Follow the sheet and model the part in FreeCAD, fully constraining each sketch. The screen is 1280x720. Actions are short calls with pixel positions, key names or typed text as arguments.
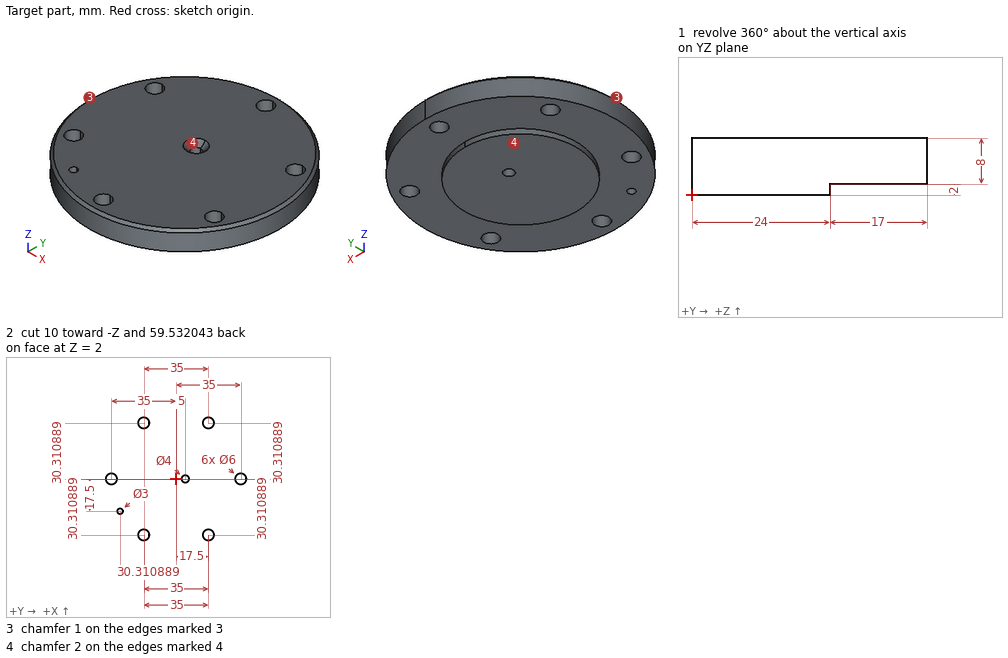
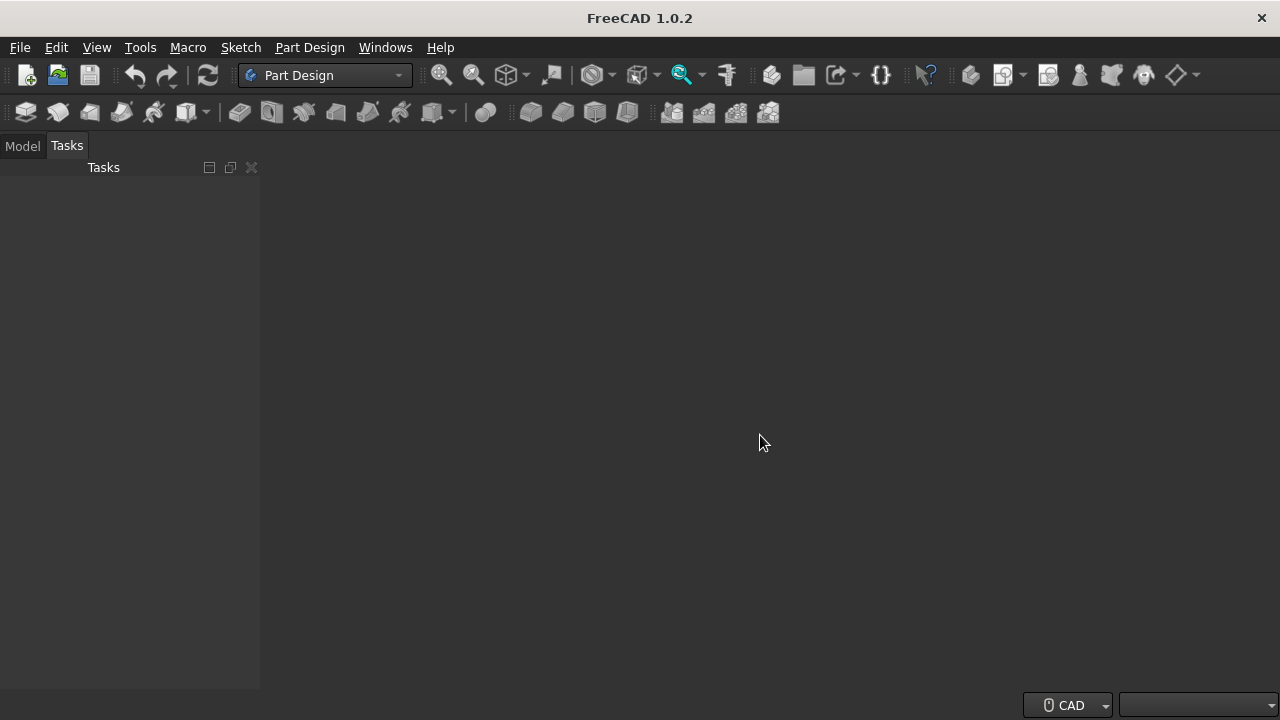
click(26, 76)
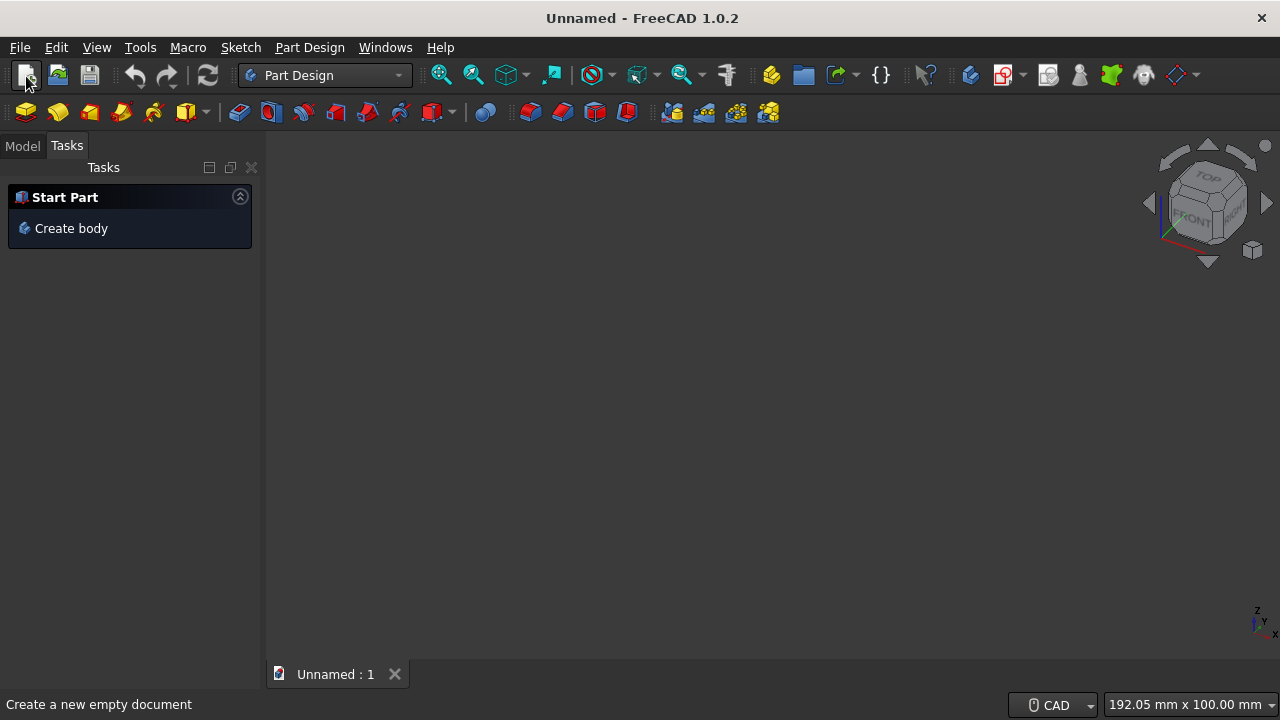
click(1004, 76)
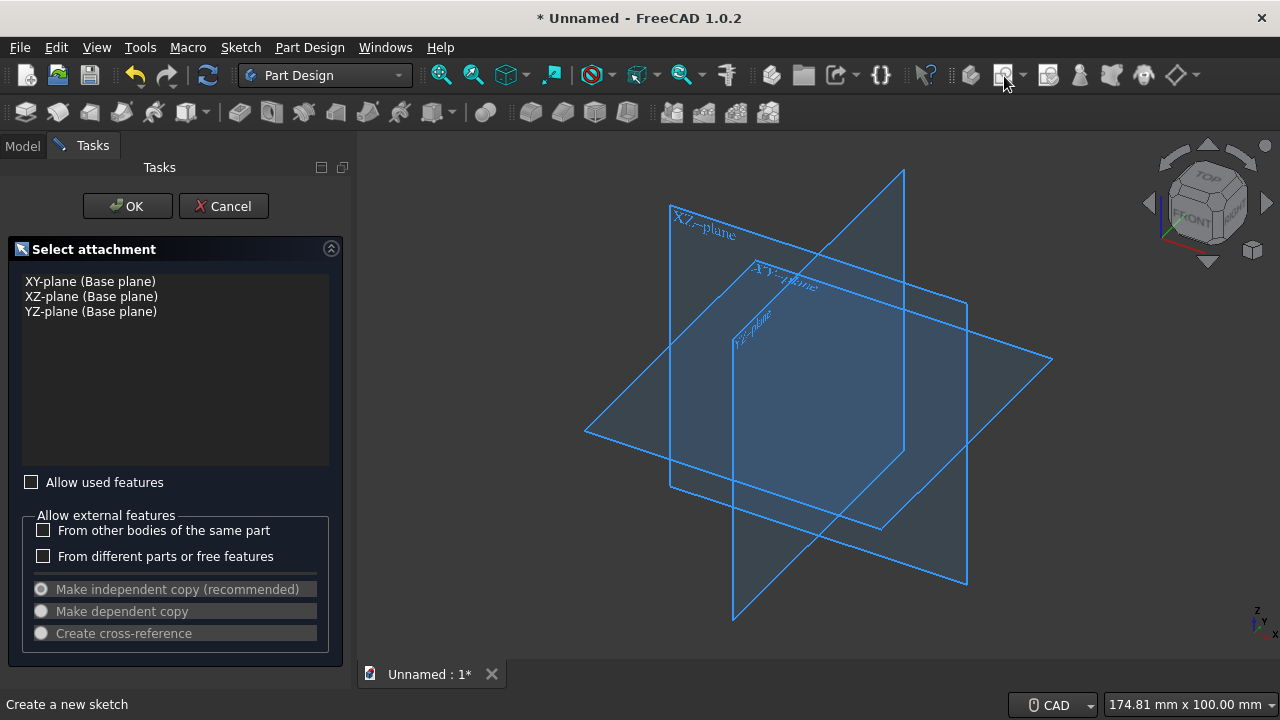
click(82, 312)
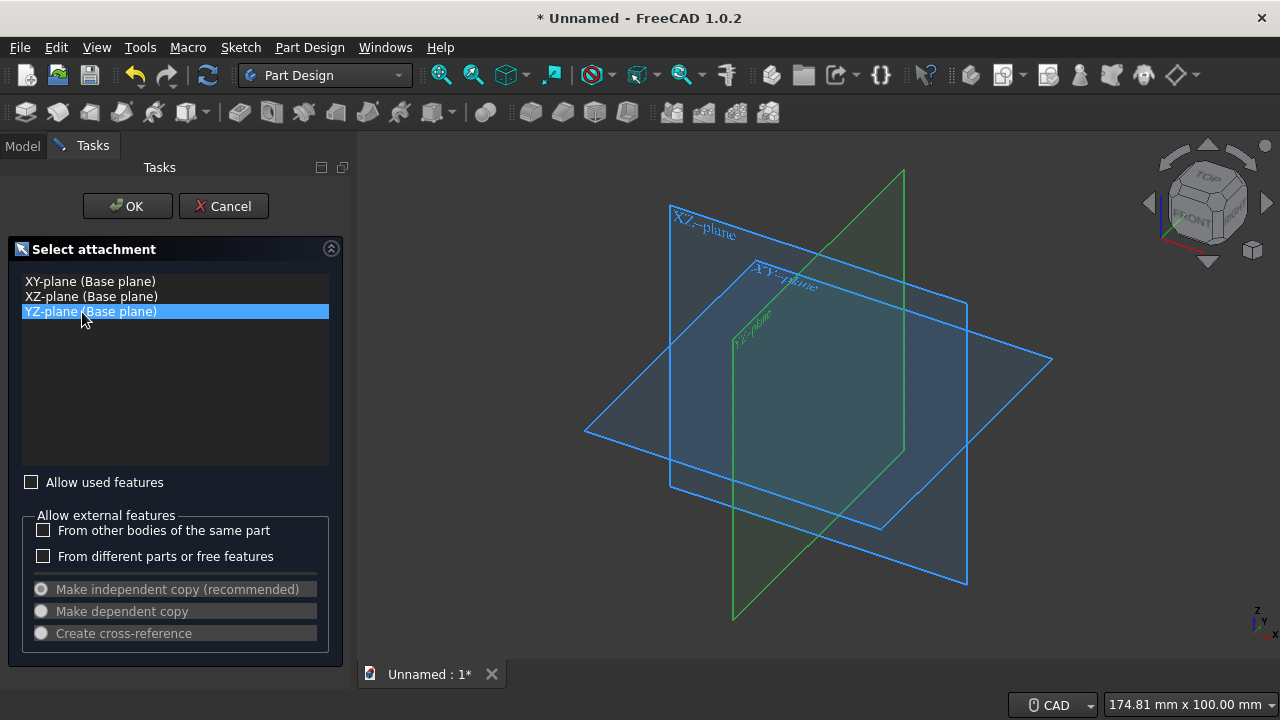
click(128, 206)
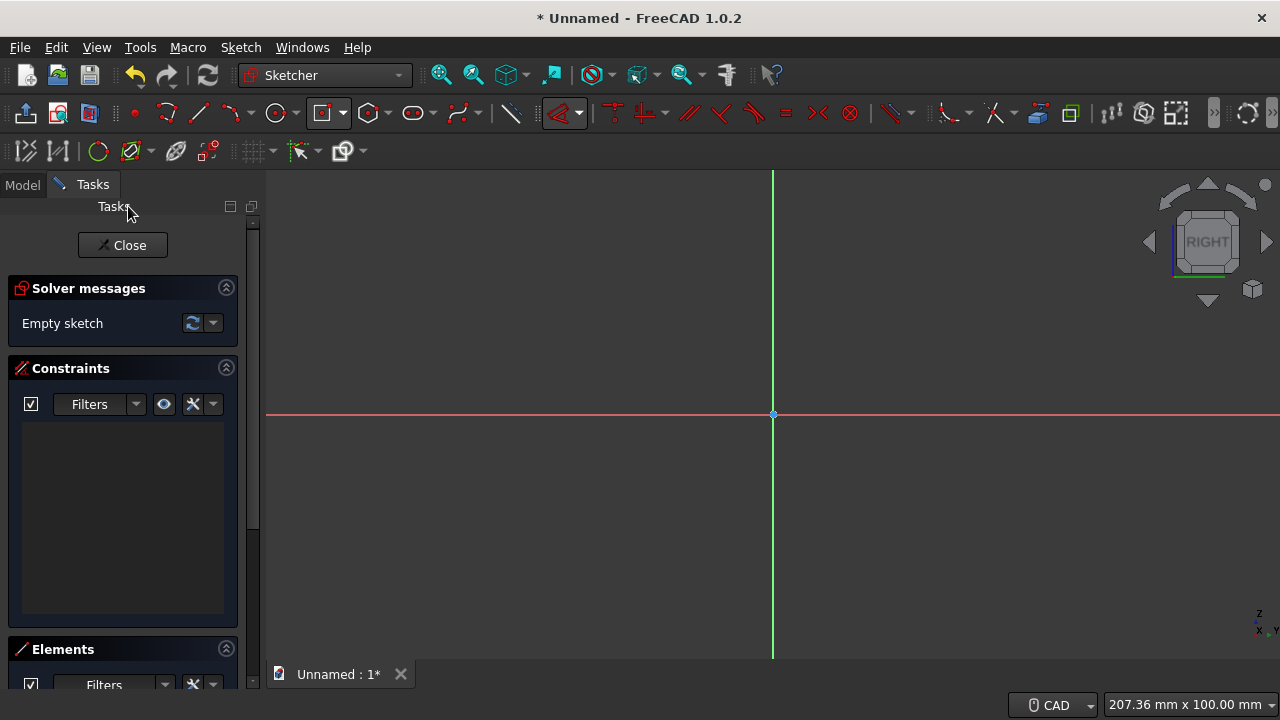
scroll(971, 376, up, 5)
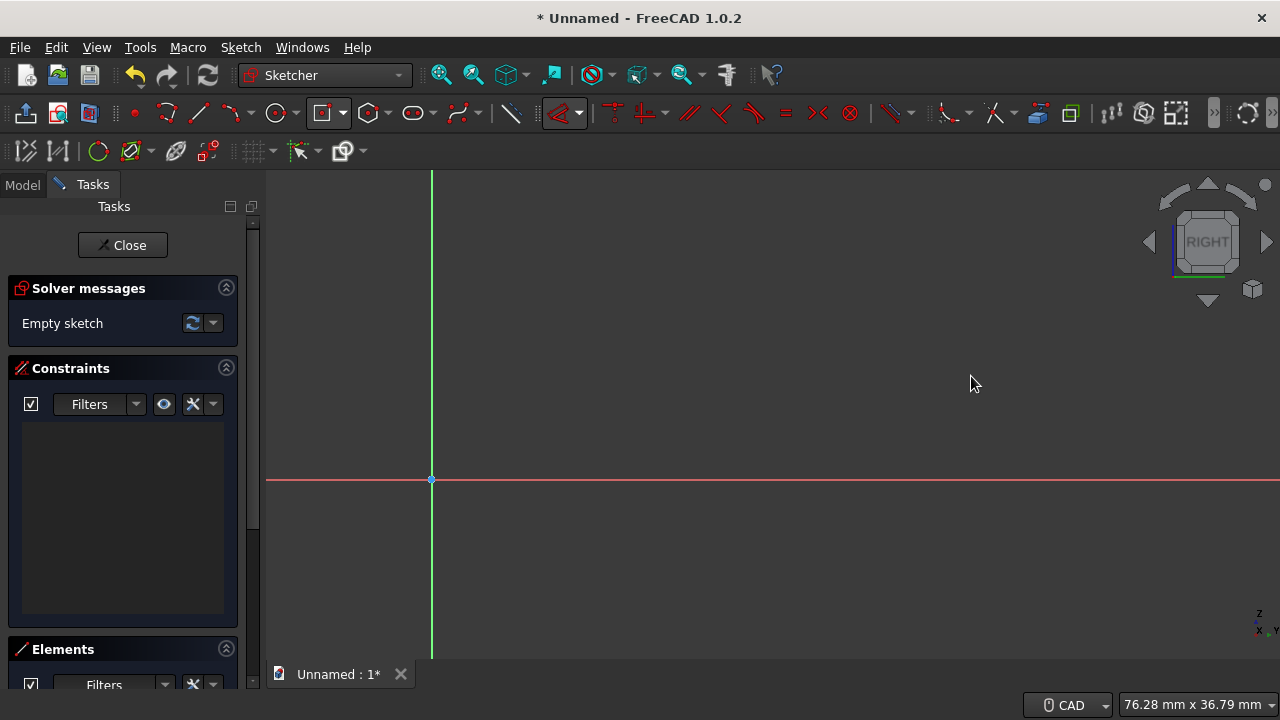
click(168, 114)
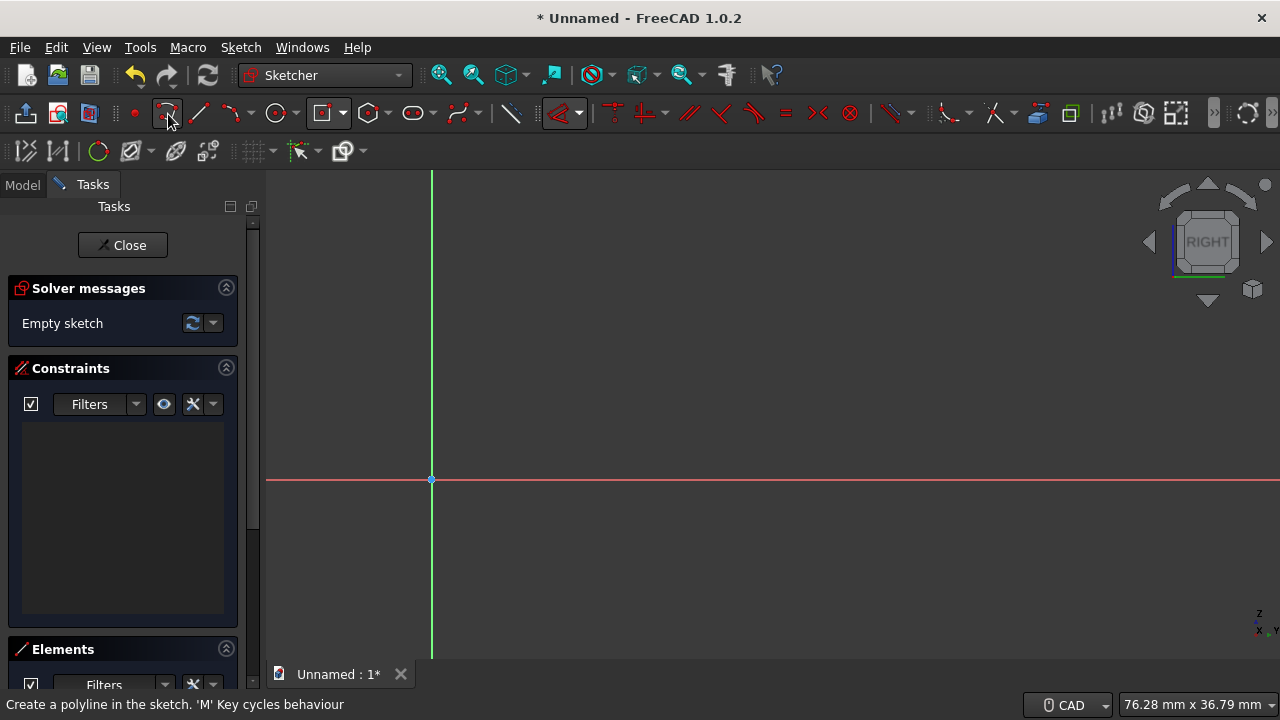
click(432, 480)
click(751, 471)
click(751, 453)
click(977, 453)
click(977, 347)
click(441, 347)
click(432, 480)
key(Escape)
key(Escape)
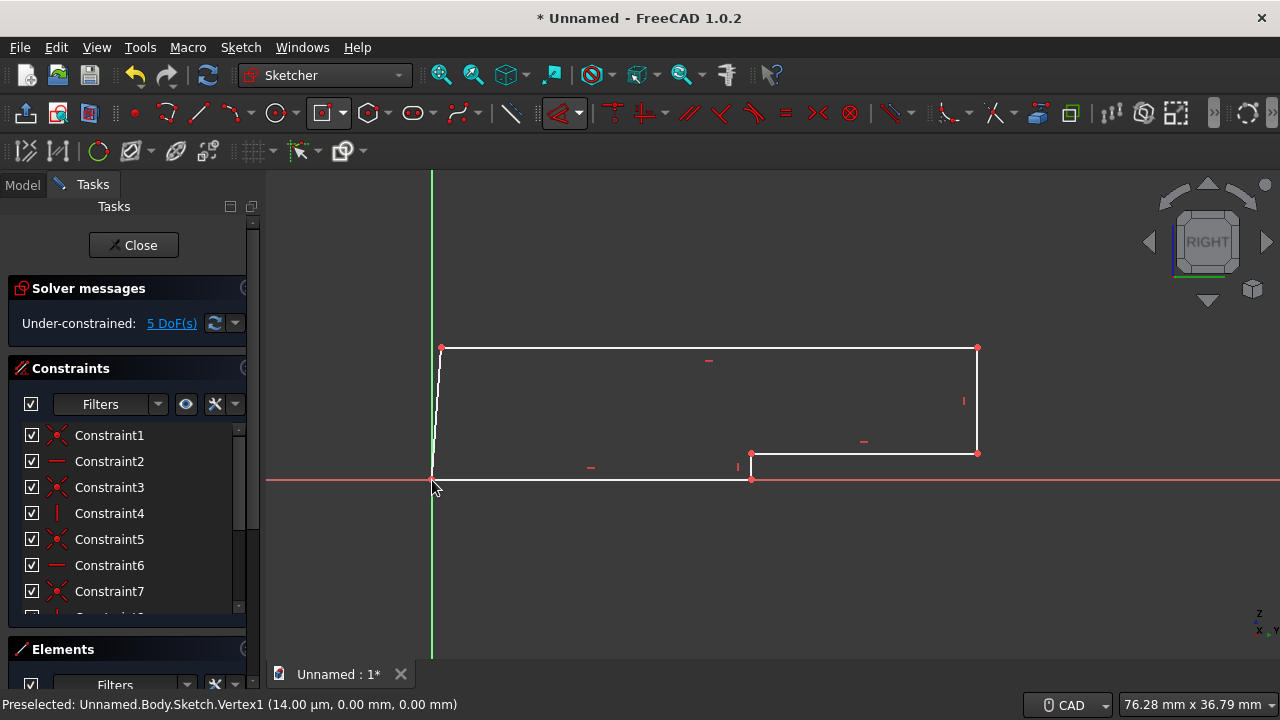
click(434, 440)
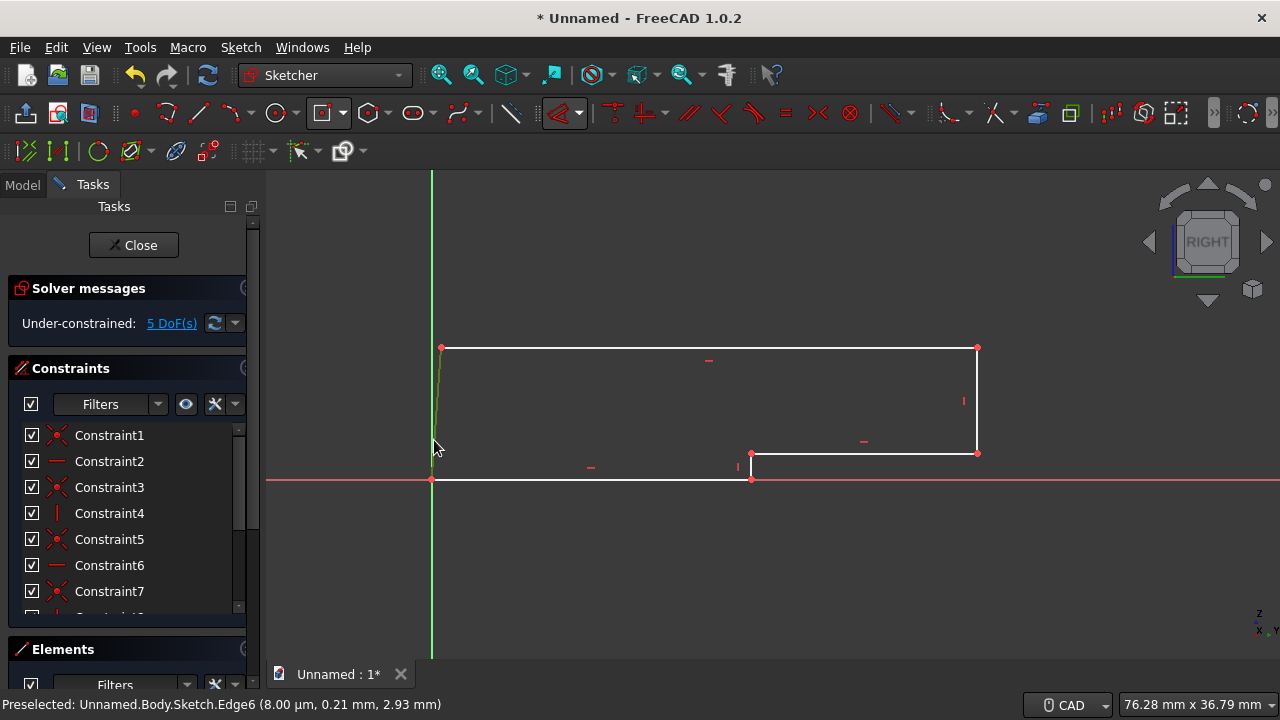
click(668, 114)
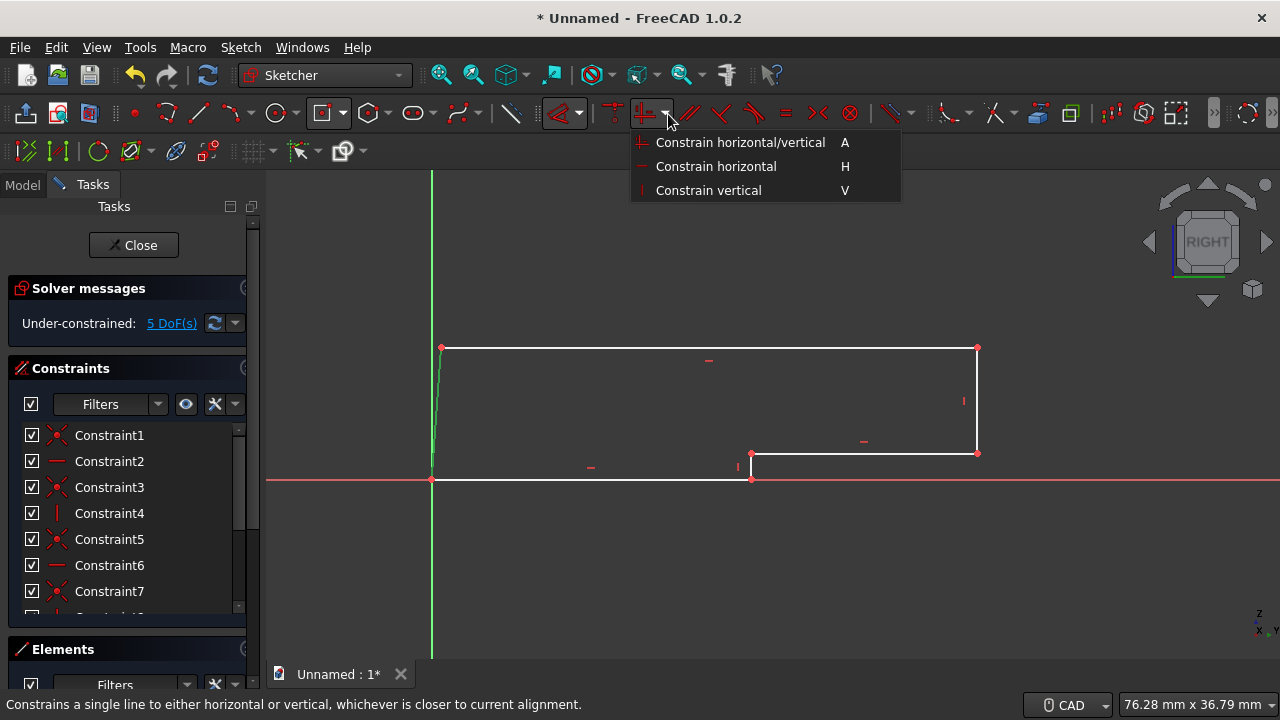
click(766, 190)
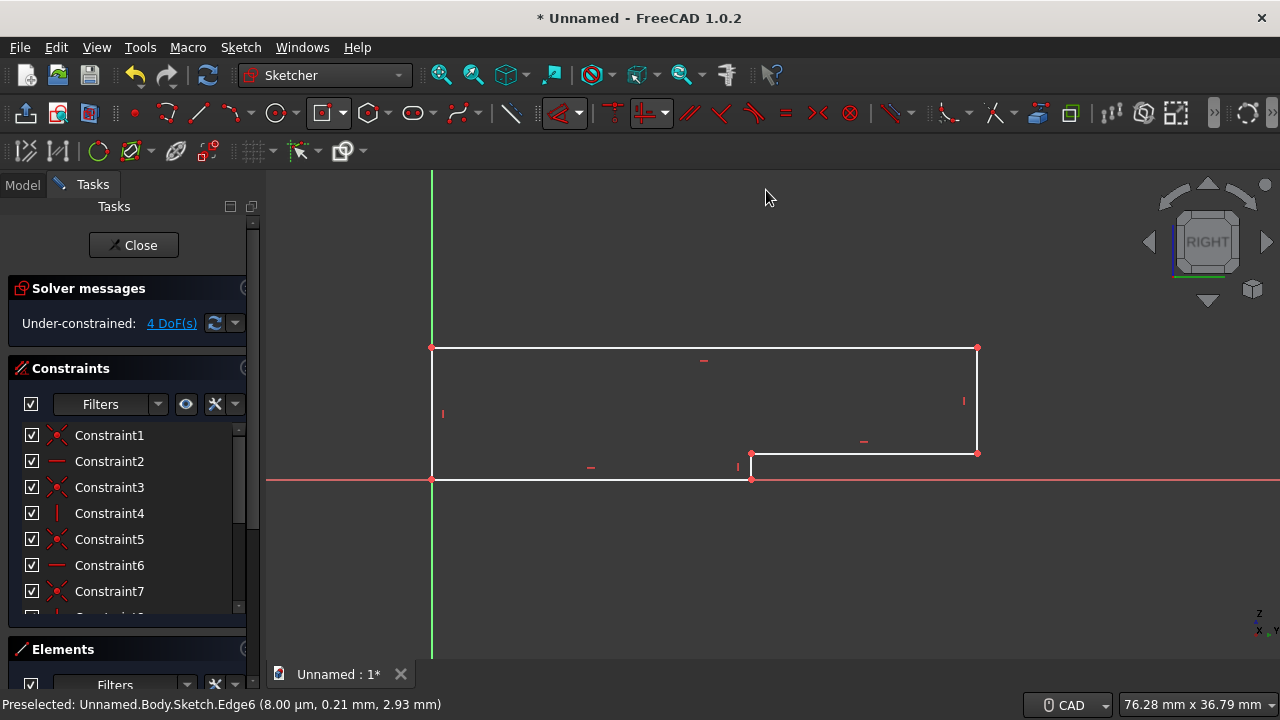
scroll(751, 470, up, 3)